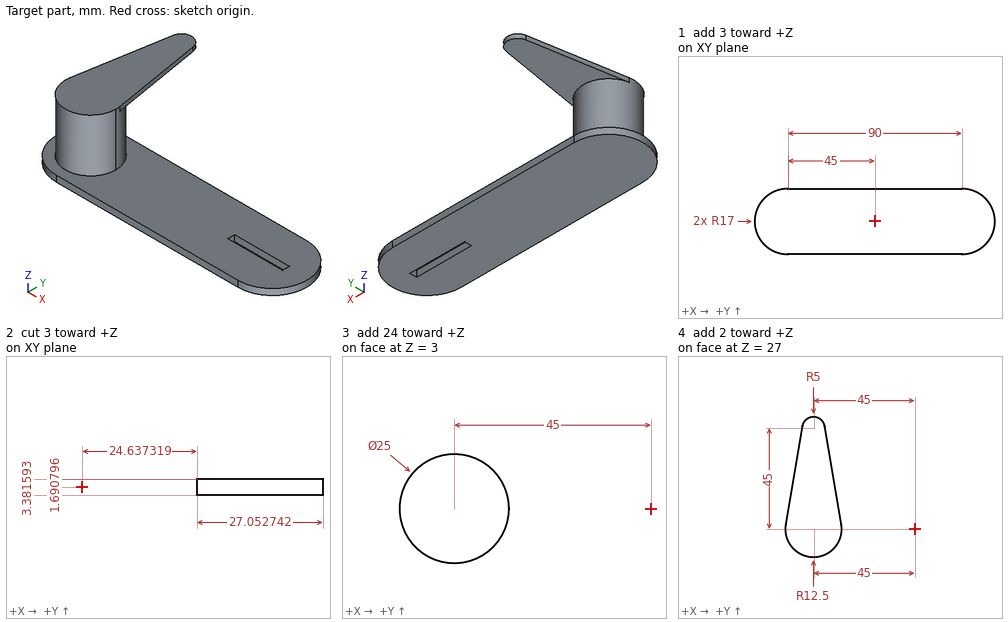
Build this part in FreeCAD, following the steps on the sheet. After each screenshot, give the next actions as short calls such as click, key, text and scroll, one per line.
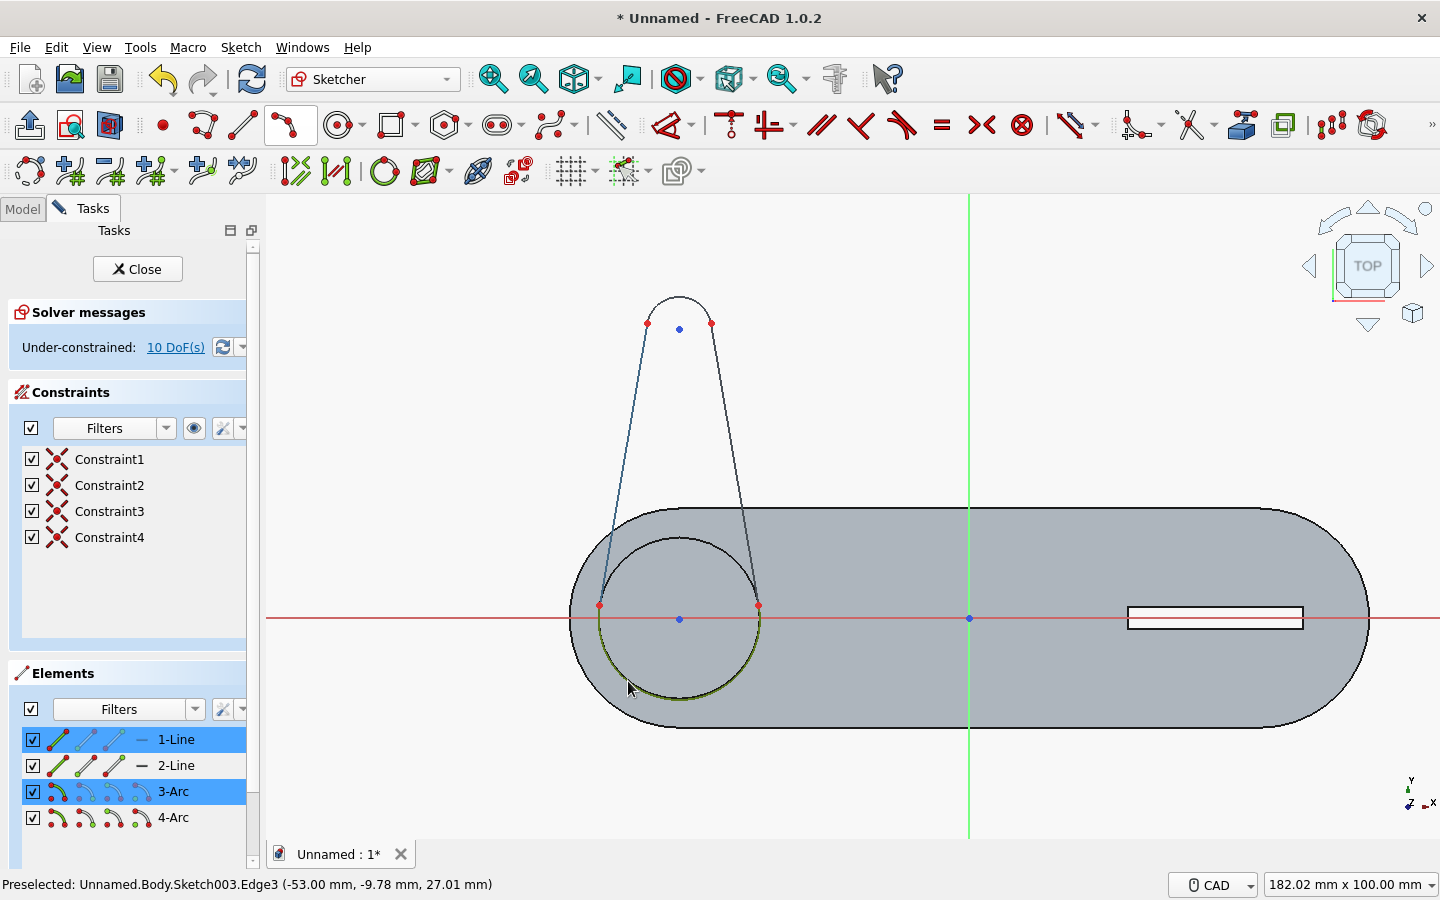
click(902, 126)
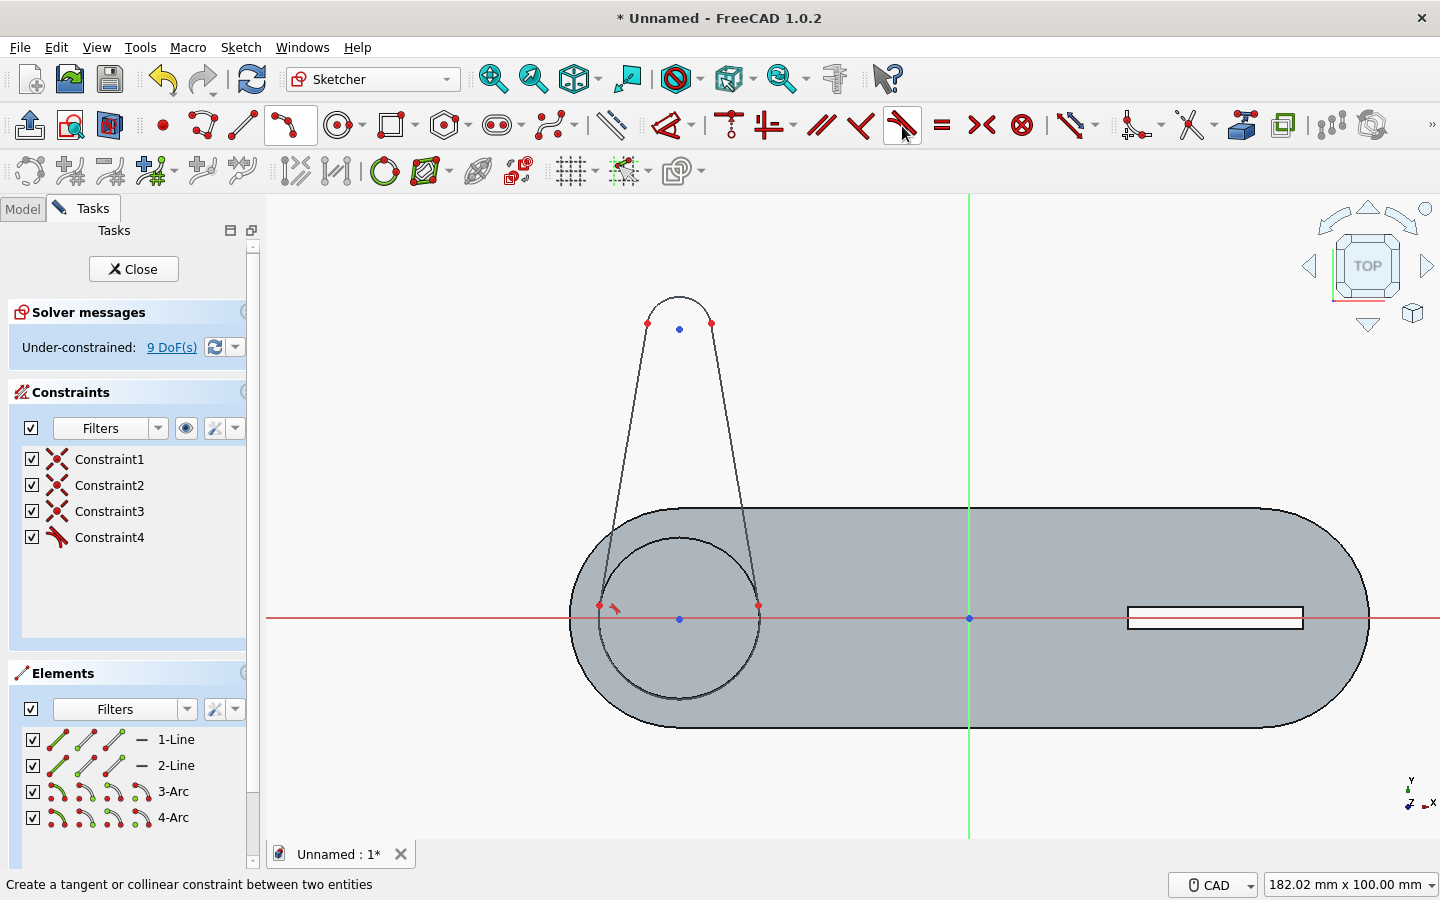
click(633, 408)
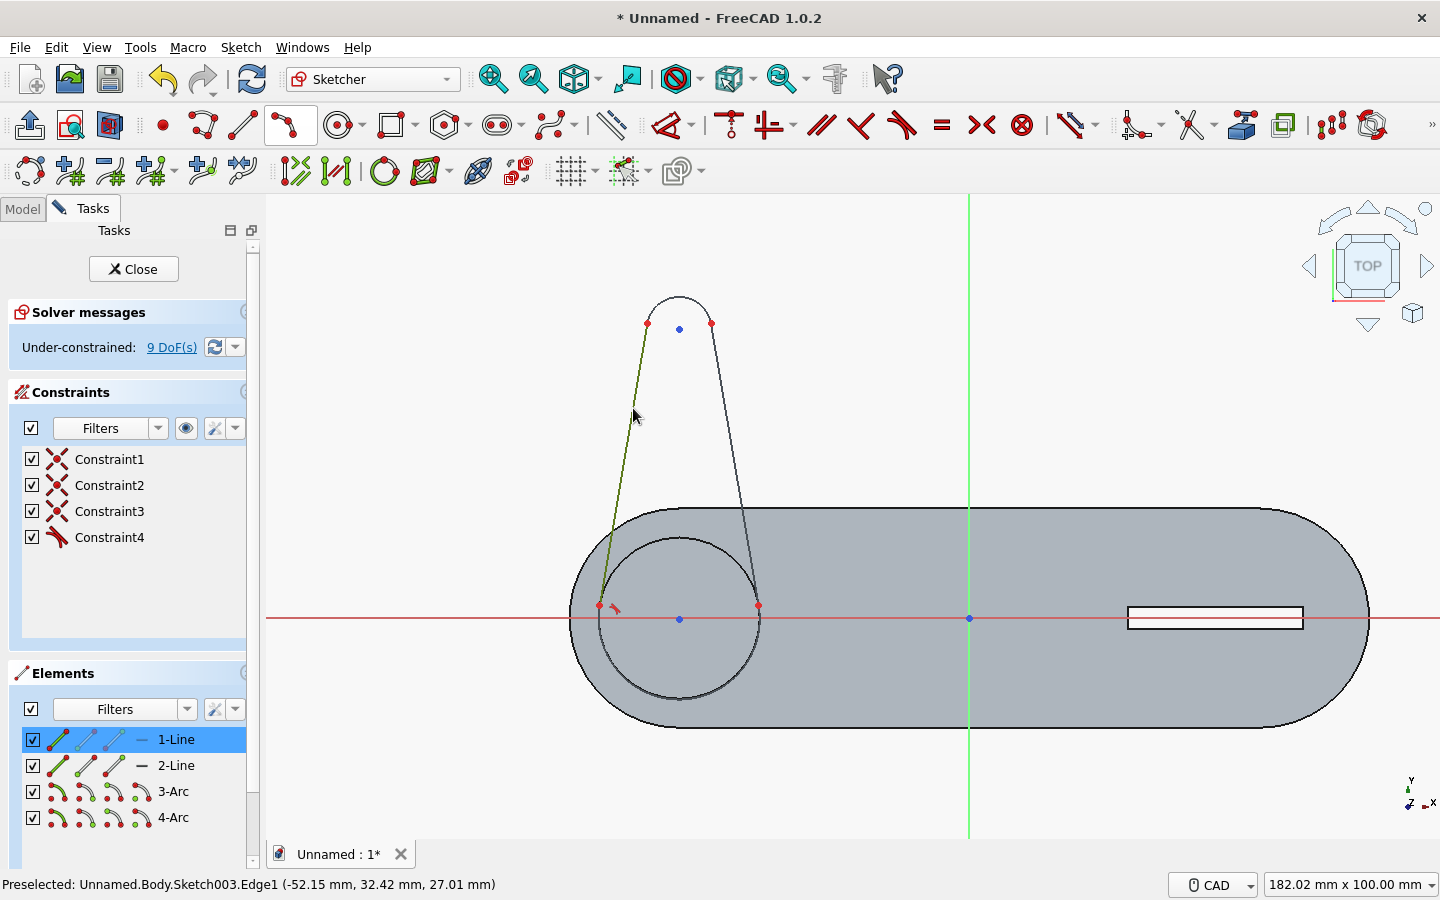
click(696, 302)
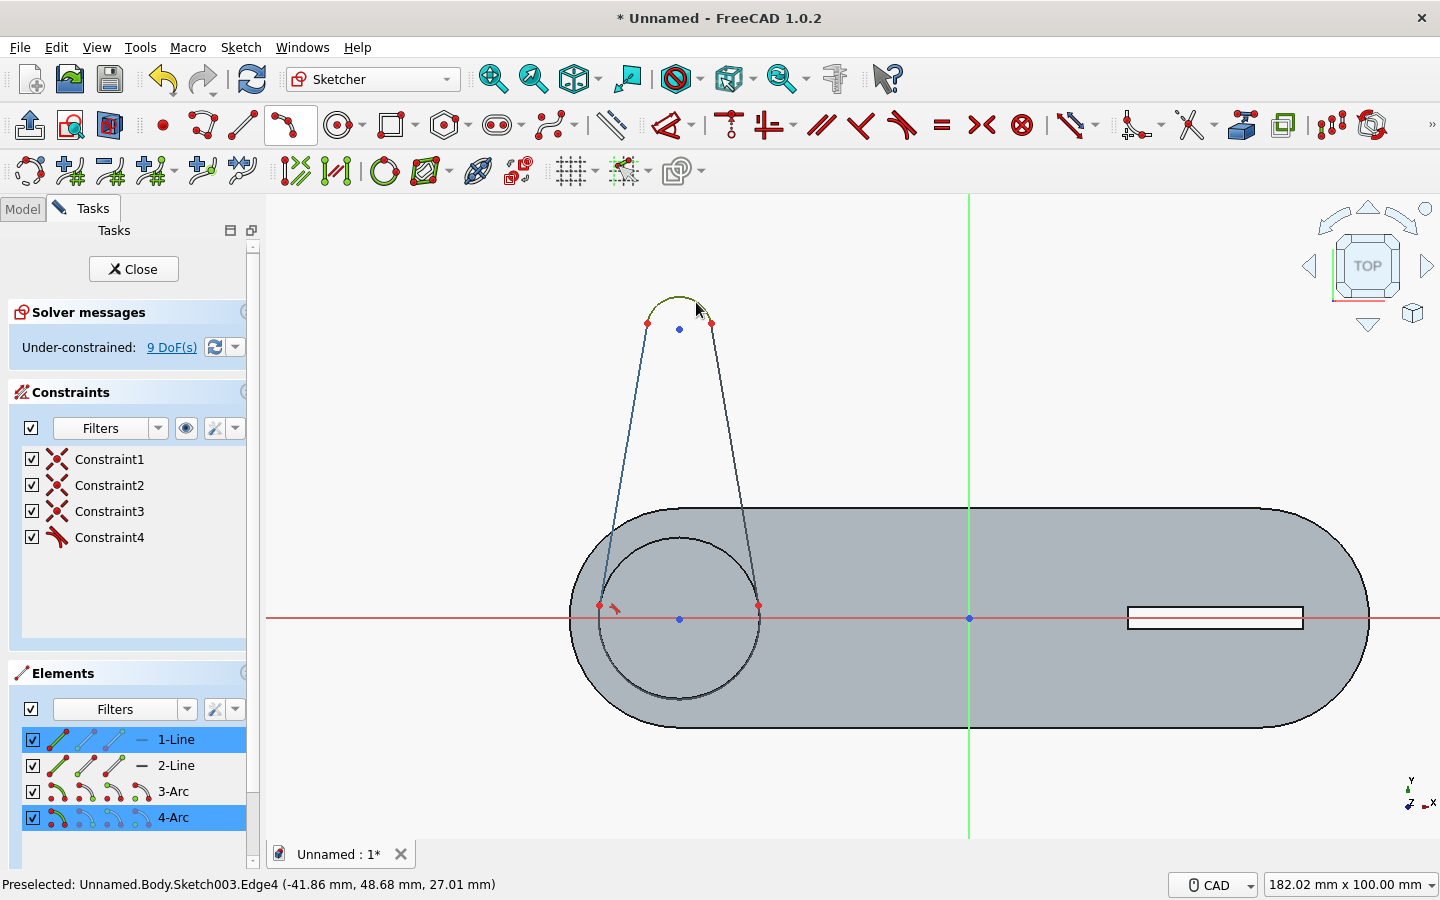
key(t)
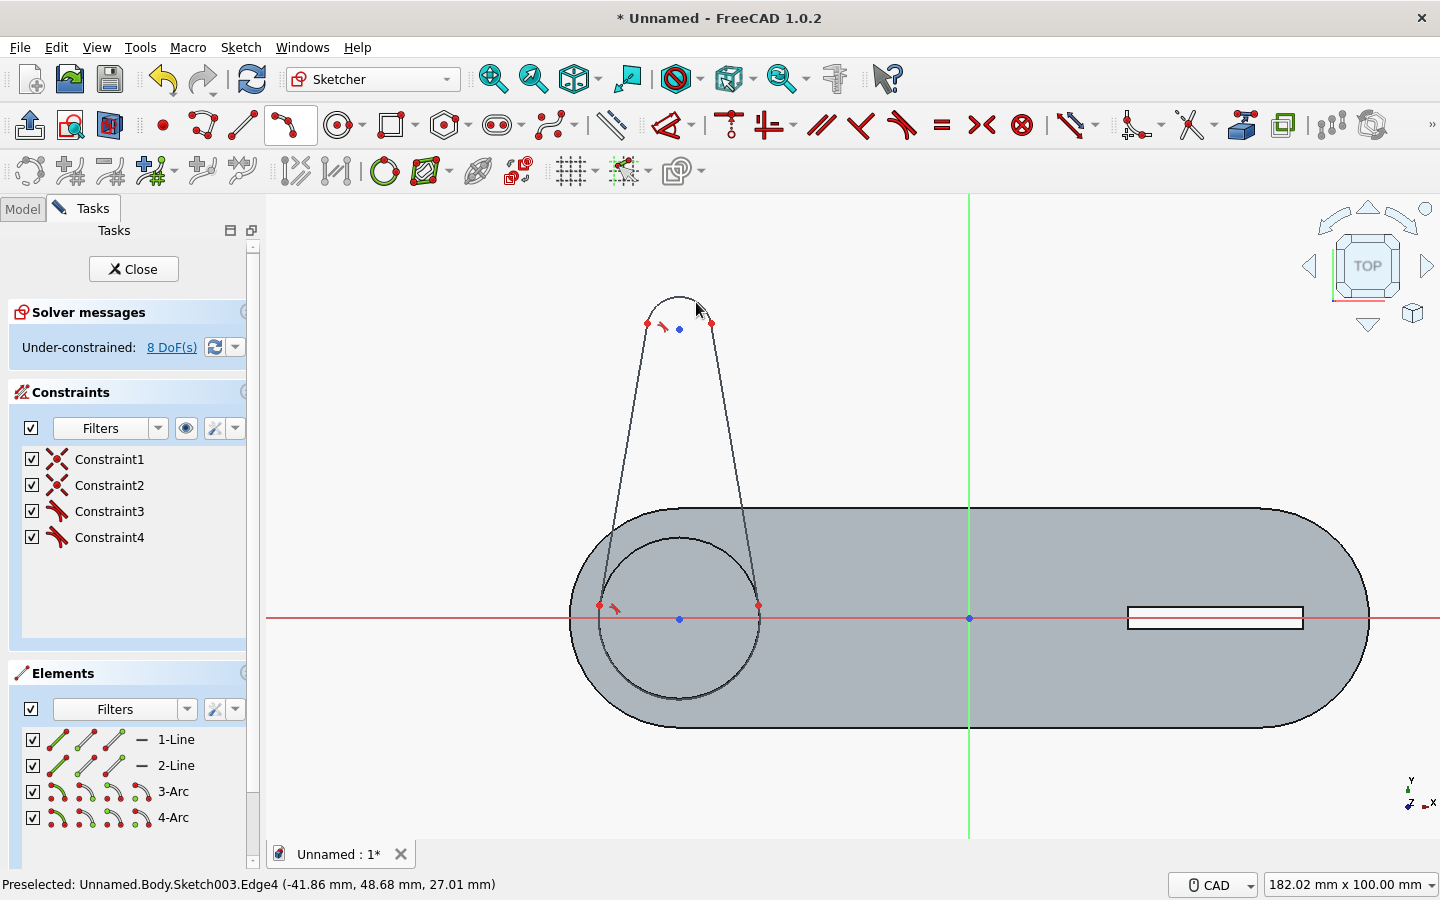
click(744, 521)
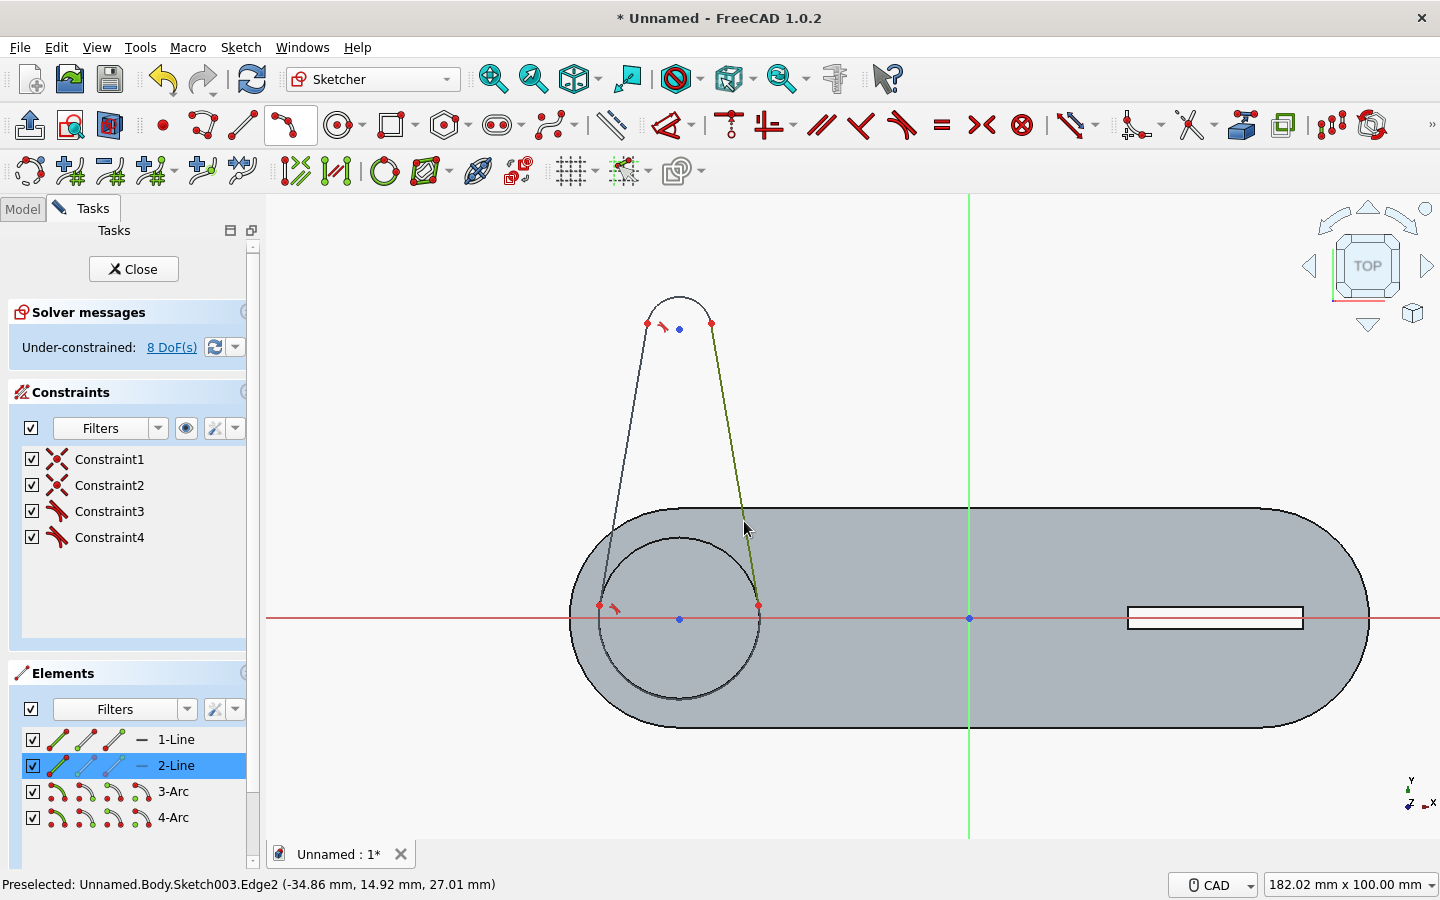
click(628, 681)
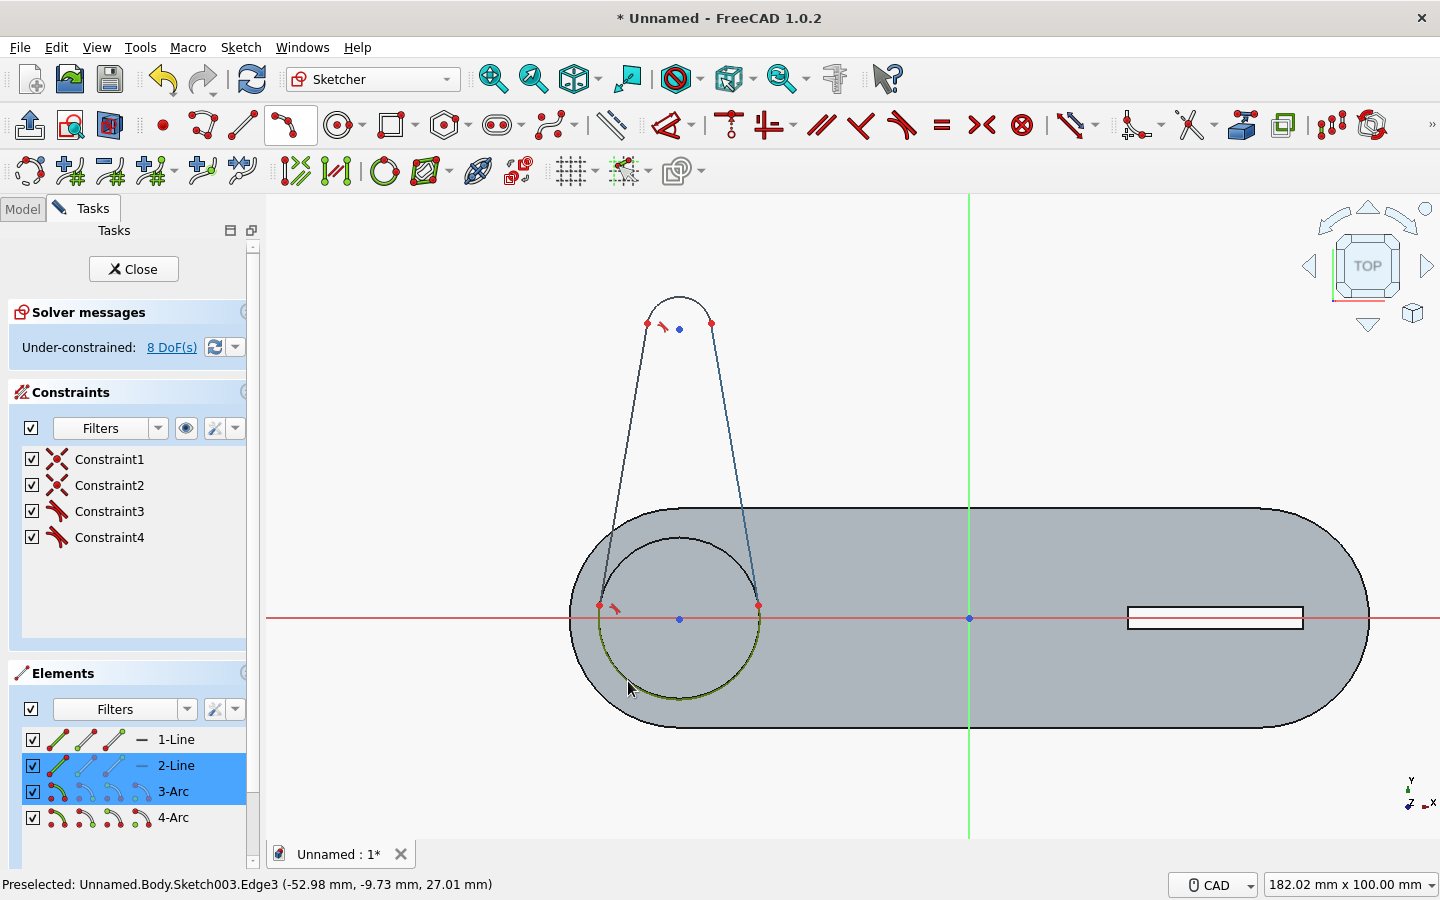
click(902, 126)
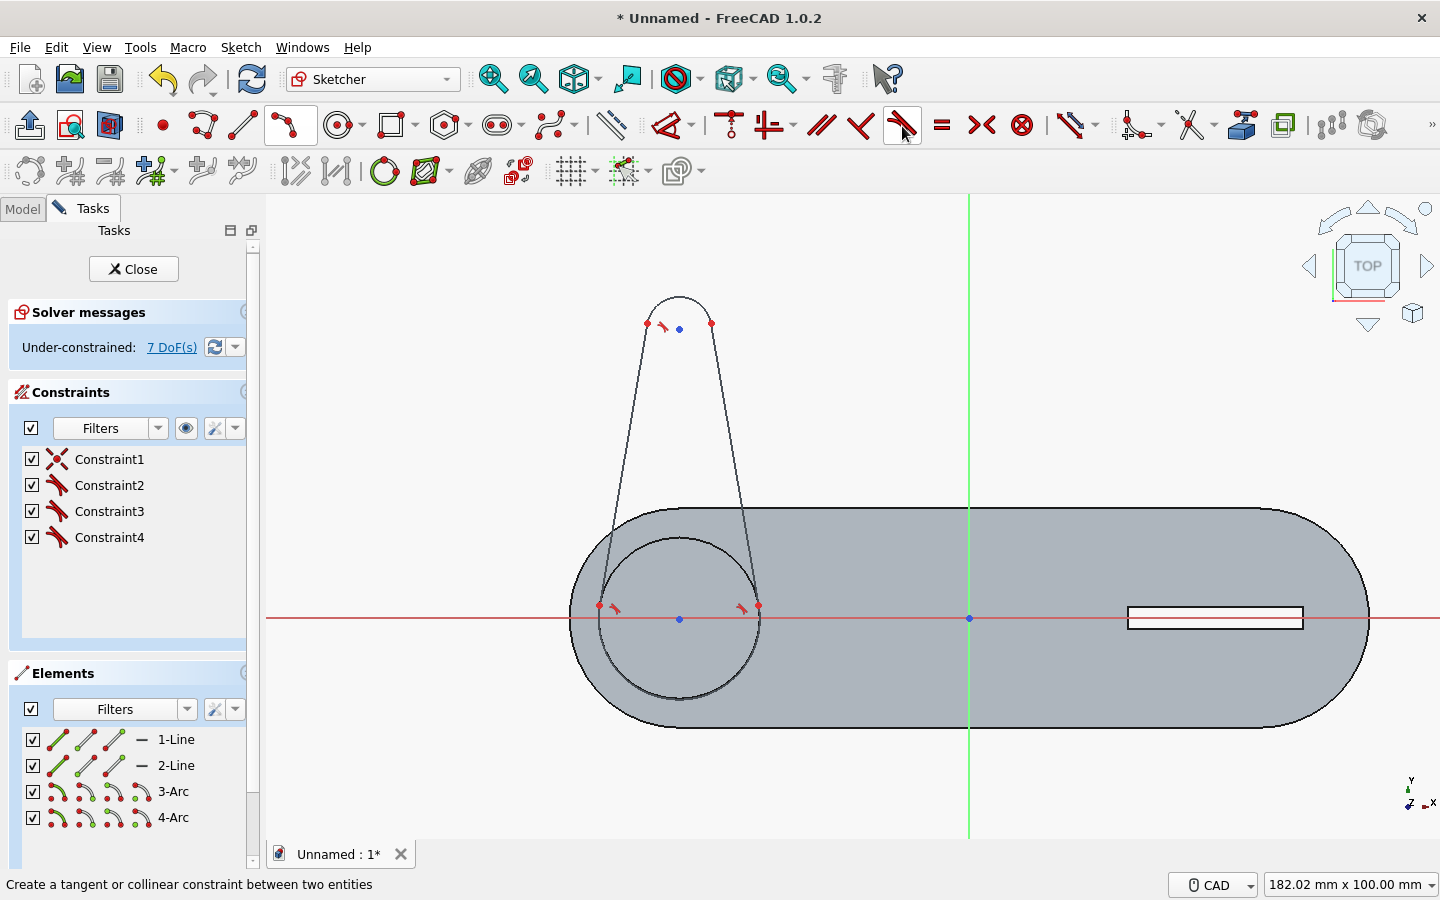
click(744, 521)